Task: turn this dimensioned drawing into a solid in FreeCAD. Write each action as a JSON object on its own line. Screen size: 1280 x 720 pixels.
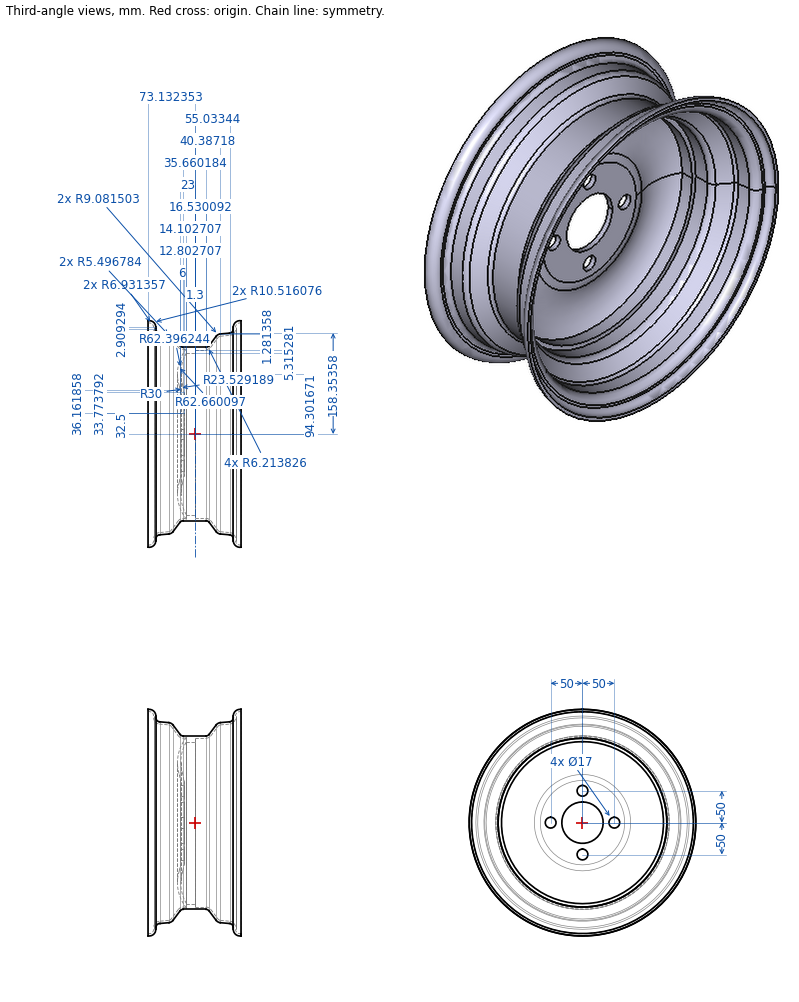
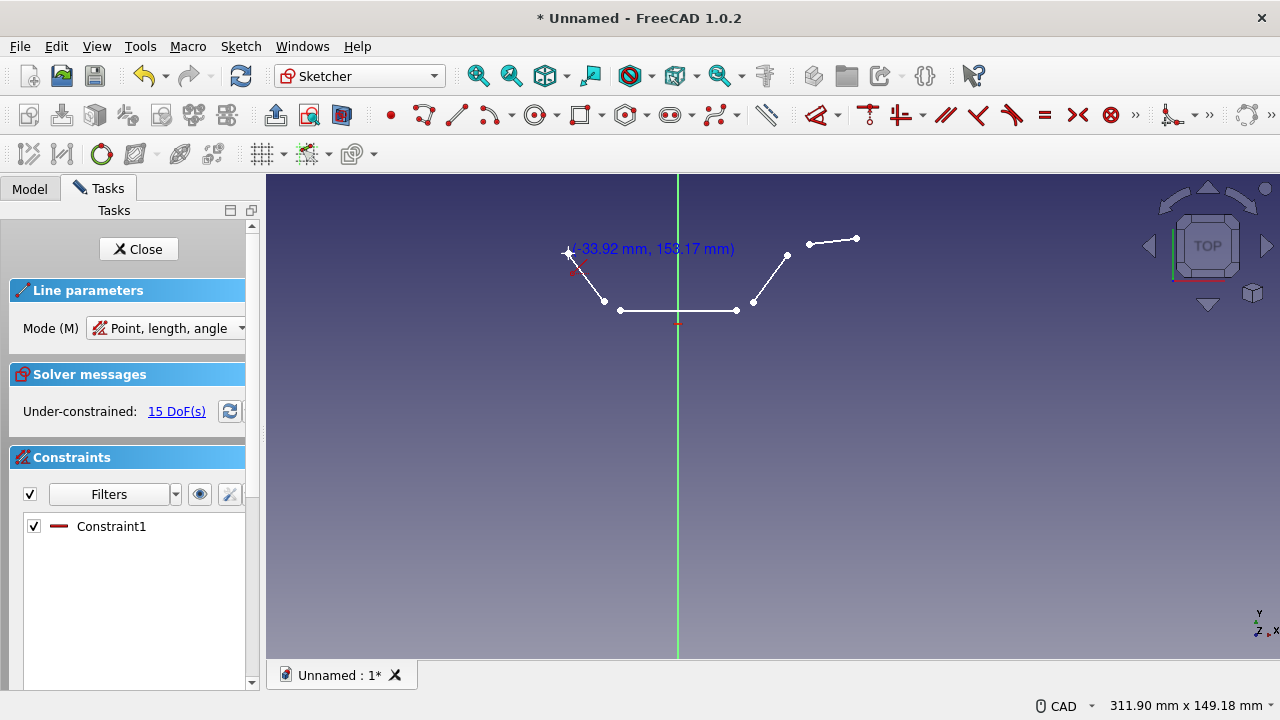
{"action": "left_click", "coordinate": [547, 241]}
{"action": "left_click", "coordinate": [499, 237]}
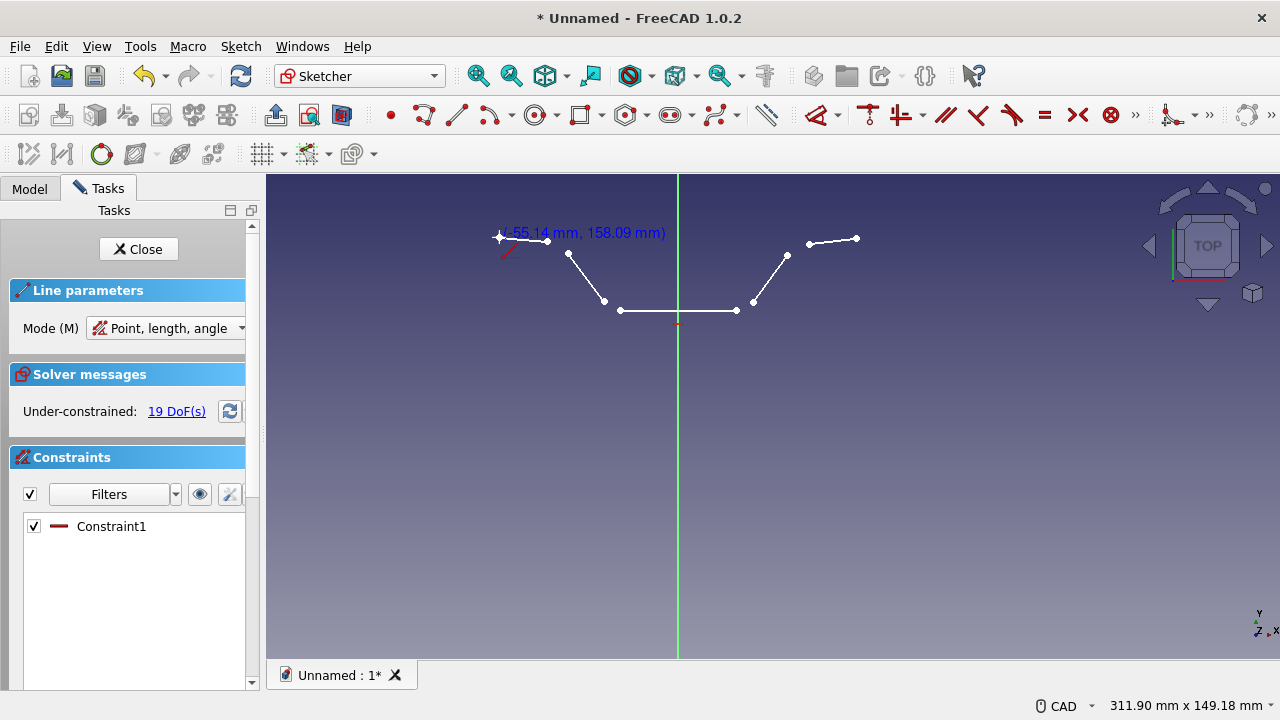
{"action": "left_click", "coordinate": [481, 217]}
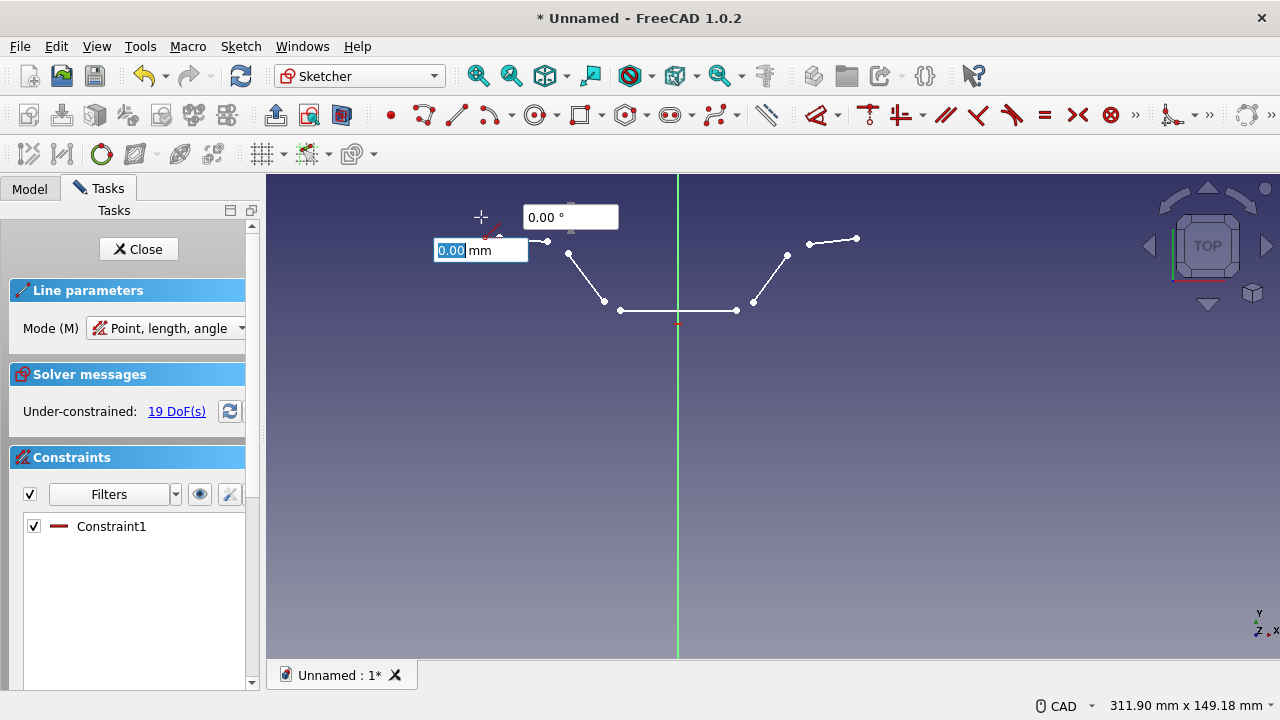
{"action": "scroll", "coordinate": [481, 208], "scroll_direction": "up", "scroll_amount": 3}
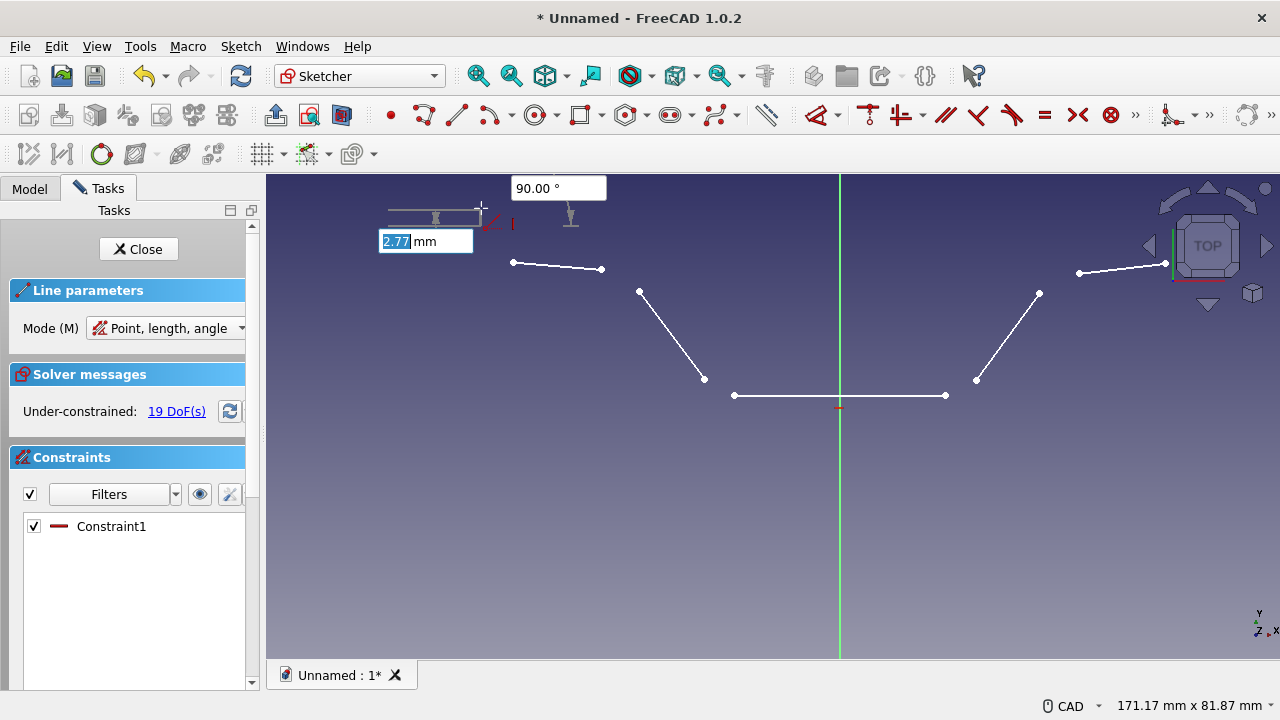
{"action": "left_click", "coordinate": [481, 207]}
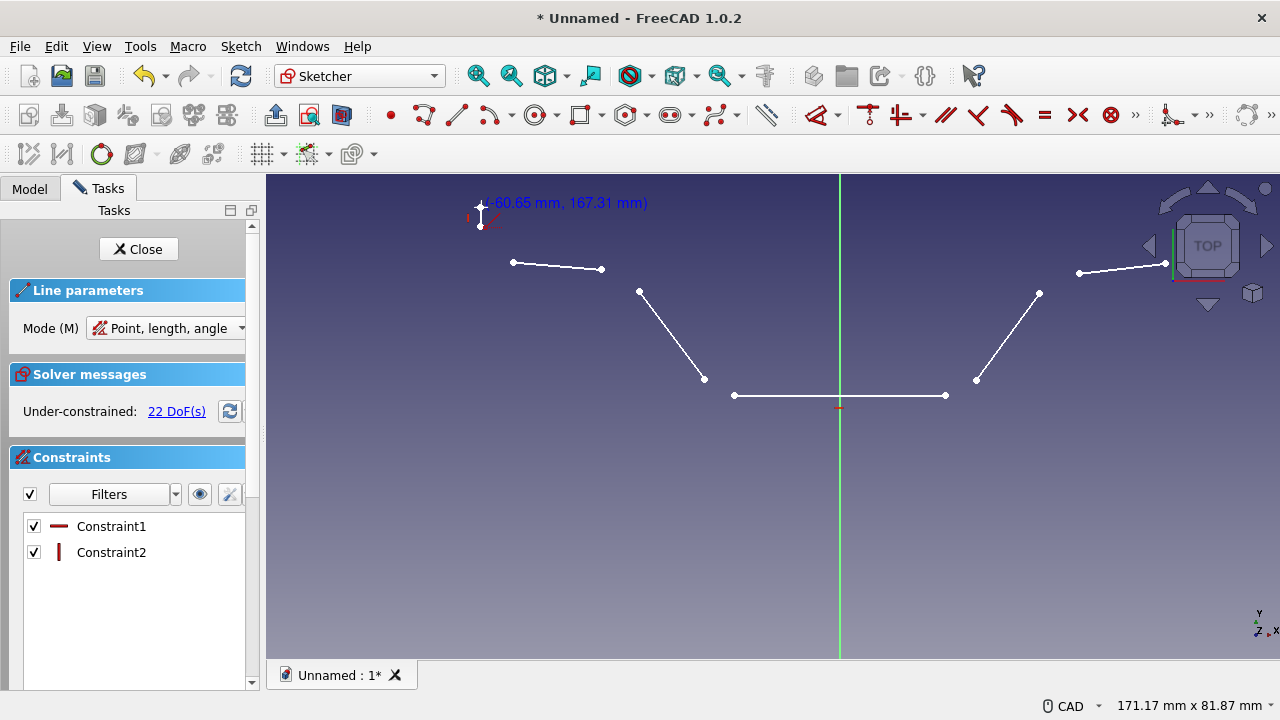
{"action": "scroll", "coordinate": [646, 306], "scroll_direction": "down", "scroll_amount": 6}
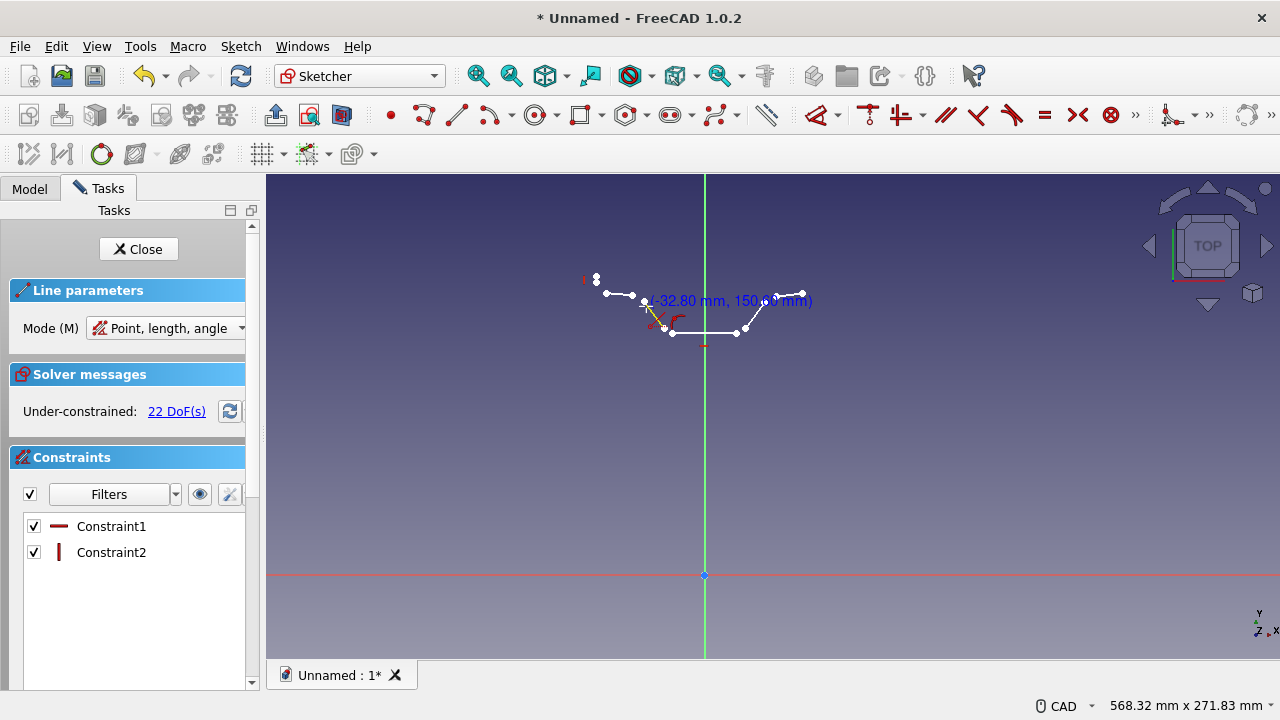
{"action": "left_click", "coordinate": [574, 258]}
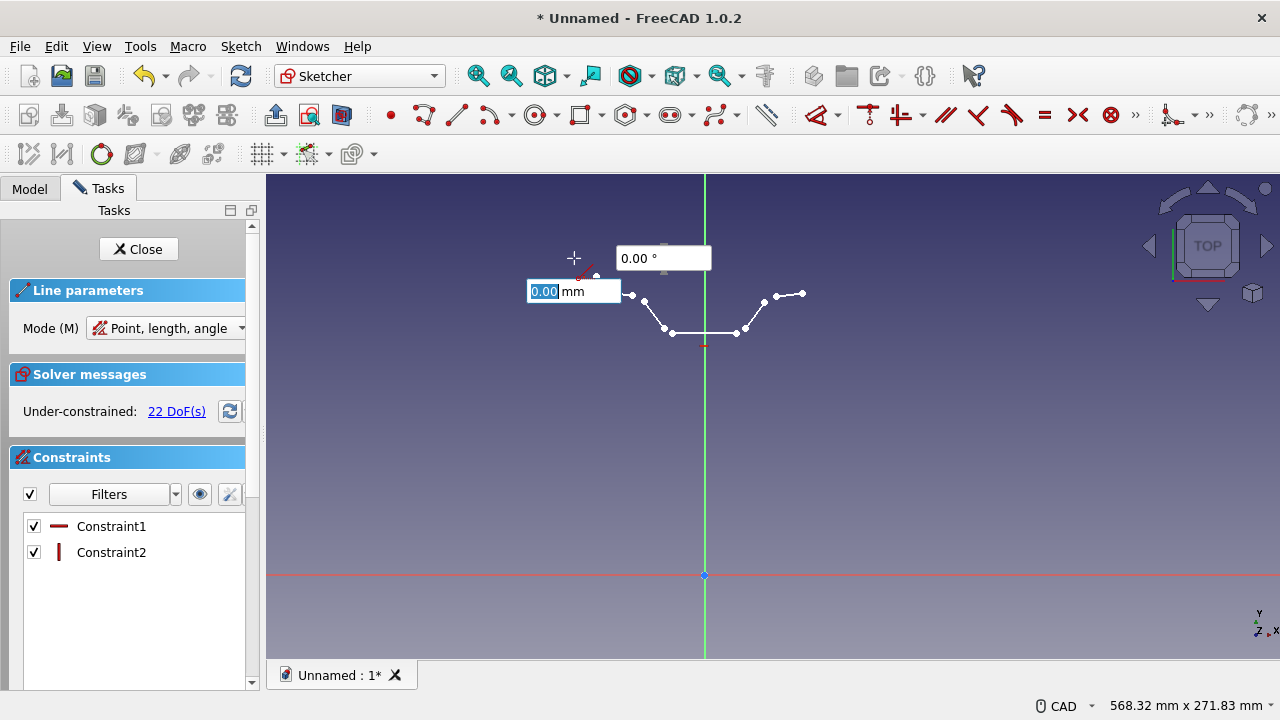
{"action": "scroll", "coordinate": [574, 265], "scroll_direction": "up", "scroll_amount": 5}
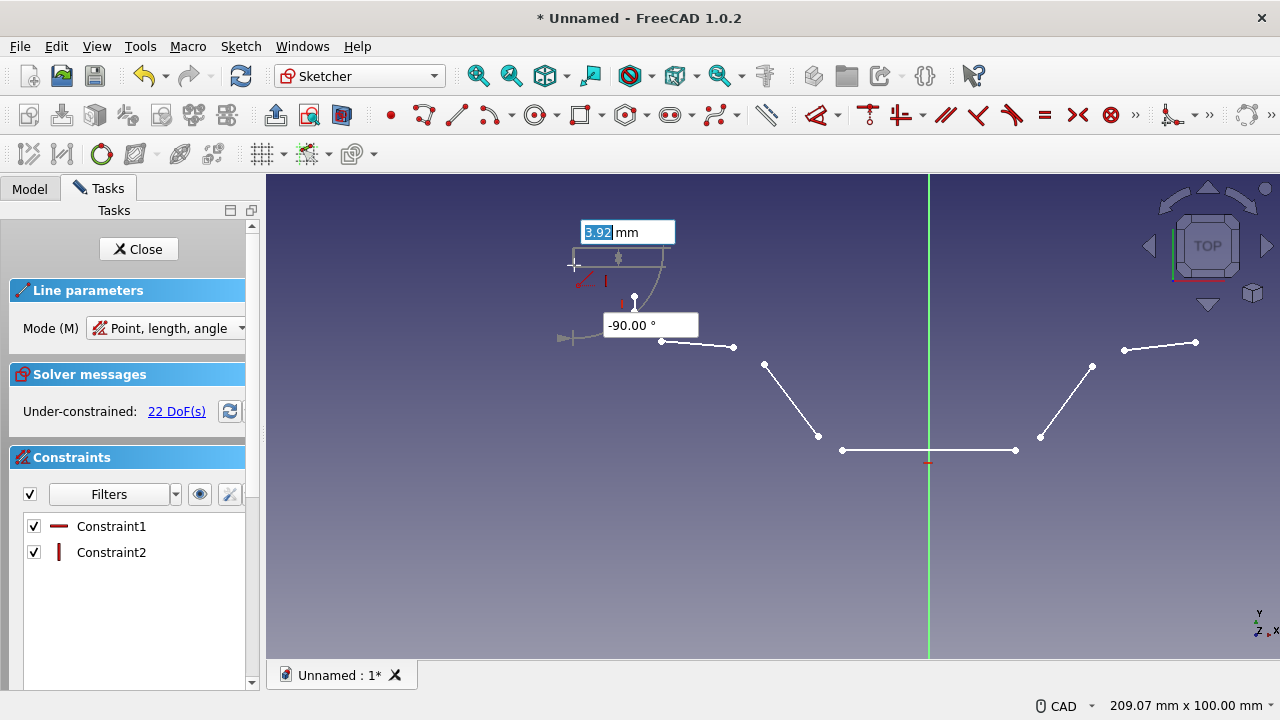
{"action": "left_click", "coordinate": [573, 263]}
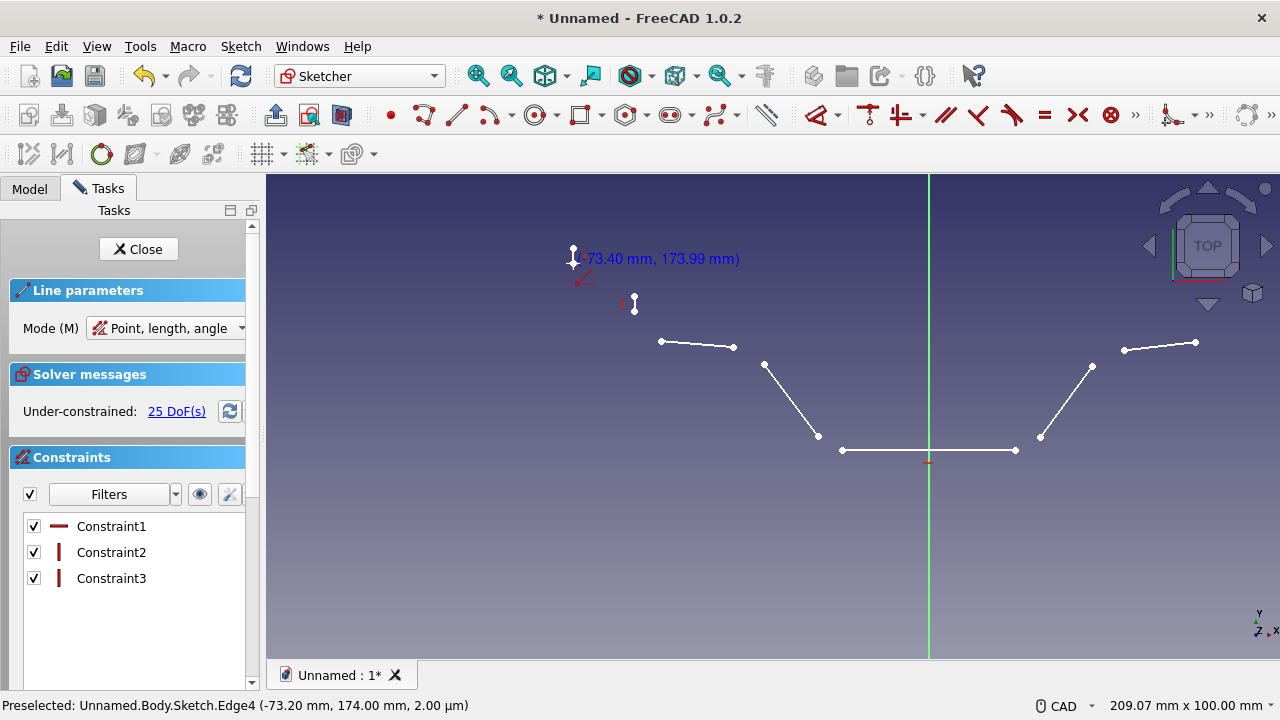
{"action": "left_click", "coordinate": [617, 296]}
{"action": "left_click", "coordinate": [617, 310]}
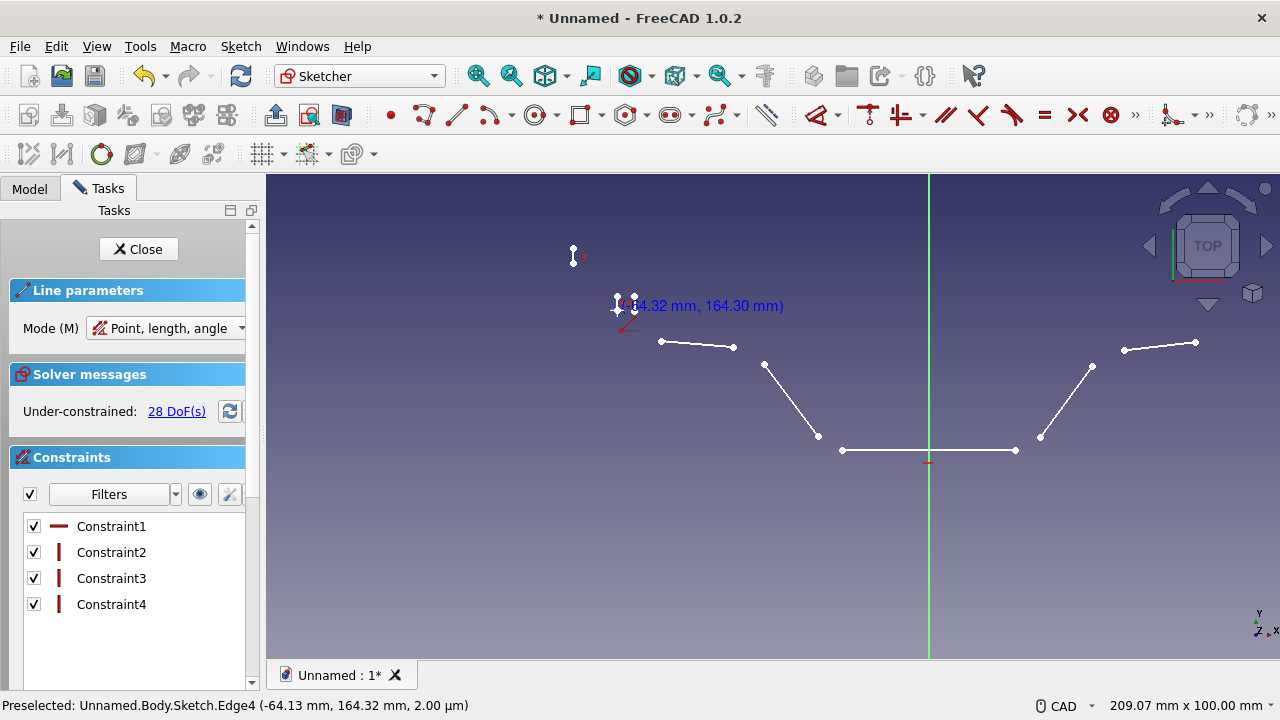
{"action": "left_click", "coordinate": [661, 357]}
{"action": "left_click", "coordinate": [732, 363]}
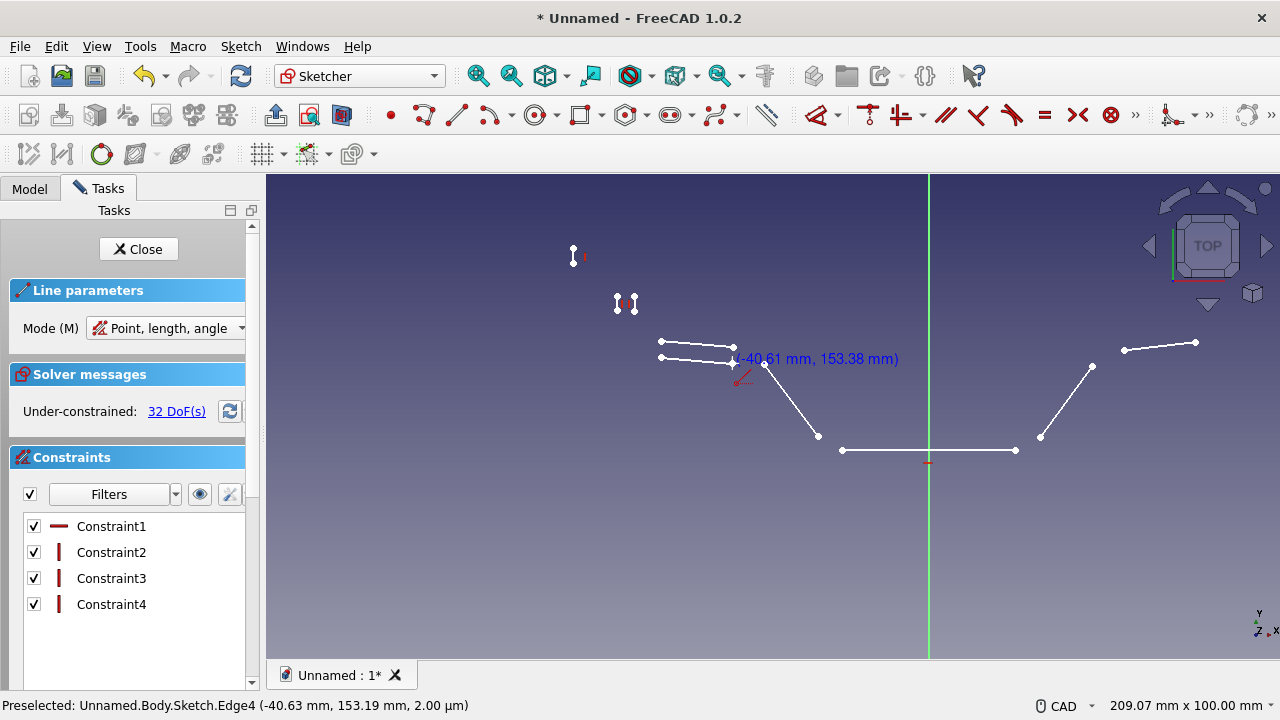
{"action": "left_click", "coordinate": [751, 374]}
{"action": "left_click", "coordinate": [804, 446]}